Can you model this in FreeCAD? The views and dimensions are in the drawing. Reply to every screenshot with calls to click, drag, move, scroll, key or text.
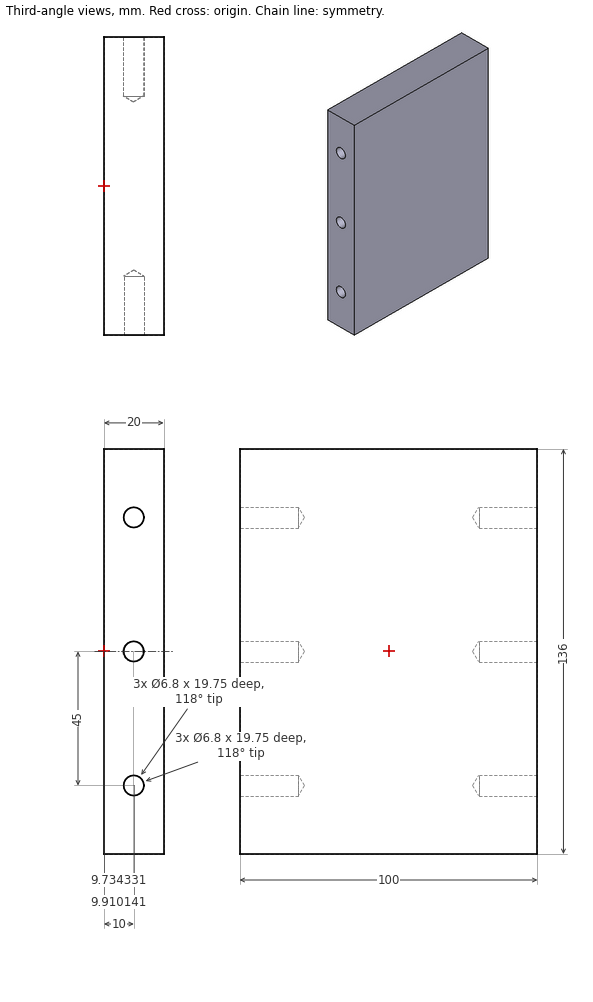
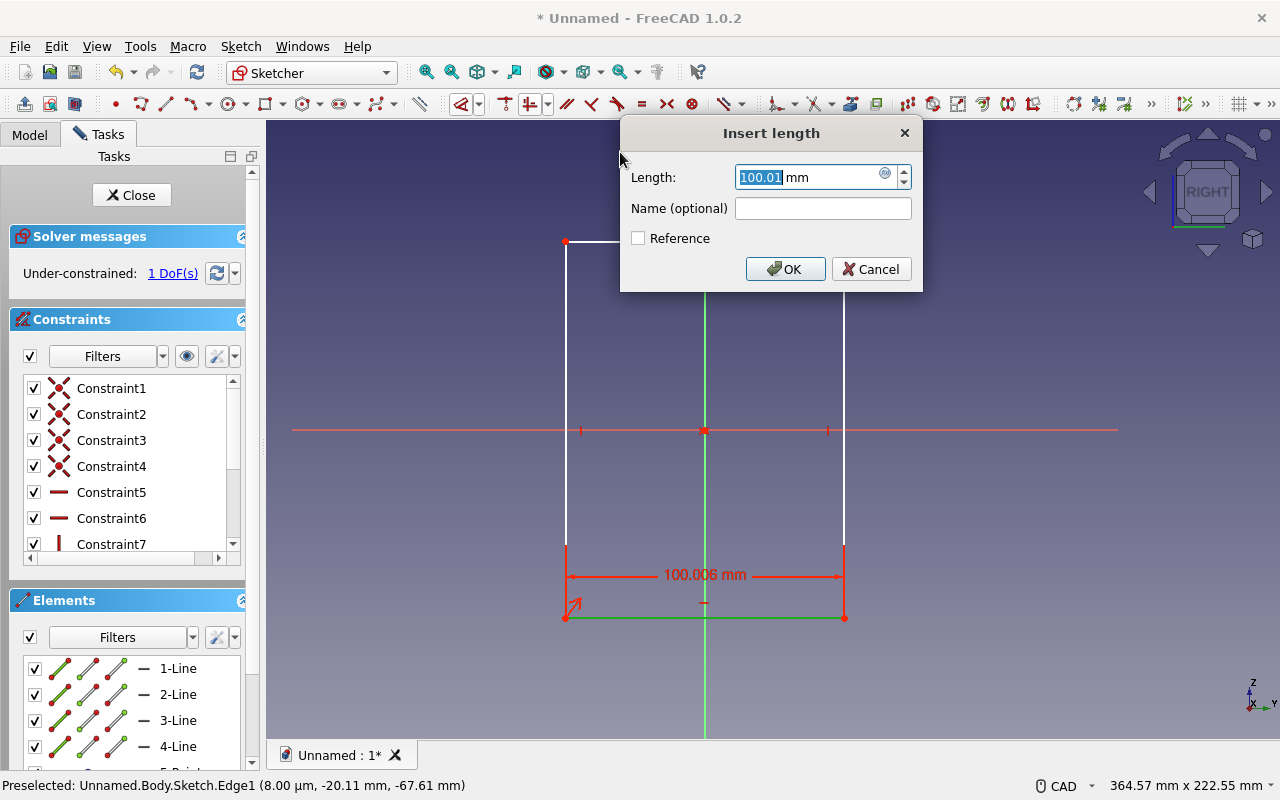
text(100)
key(Return)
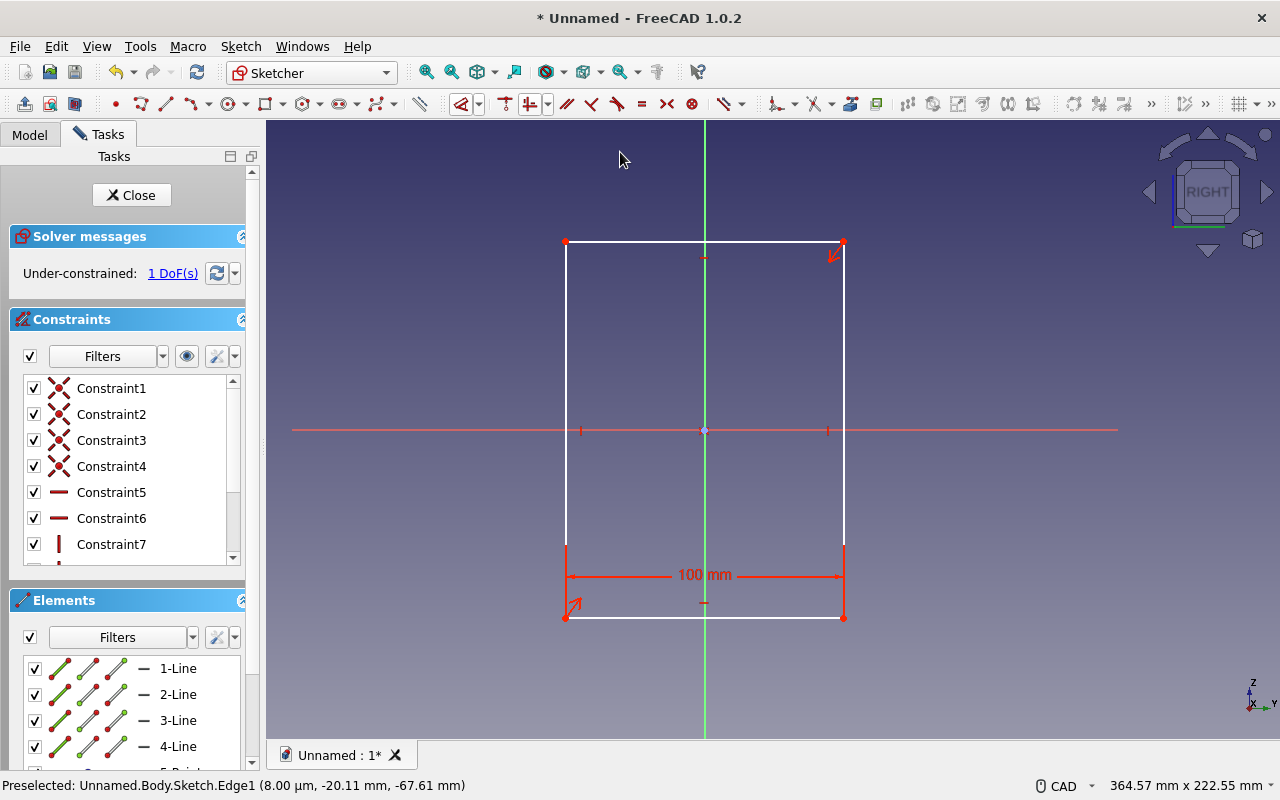
click(844, 505)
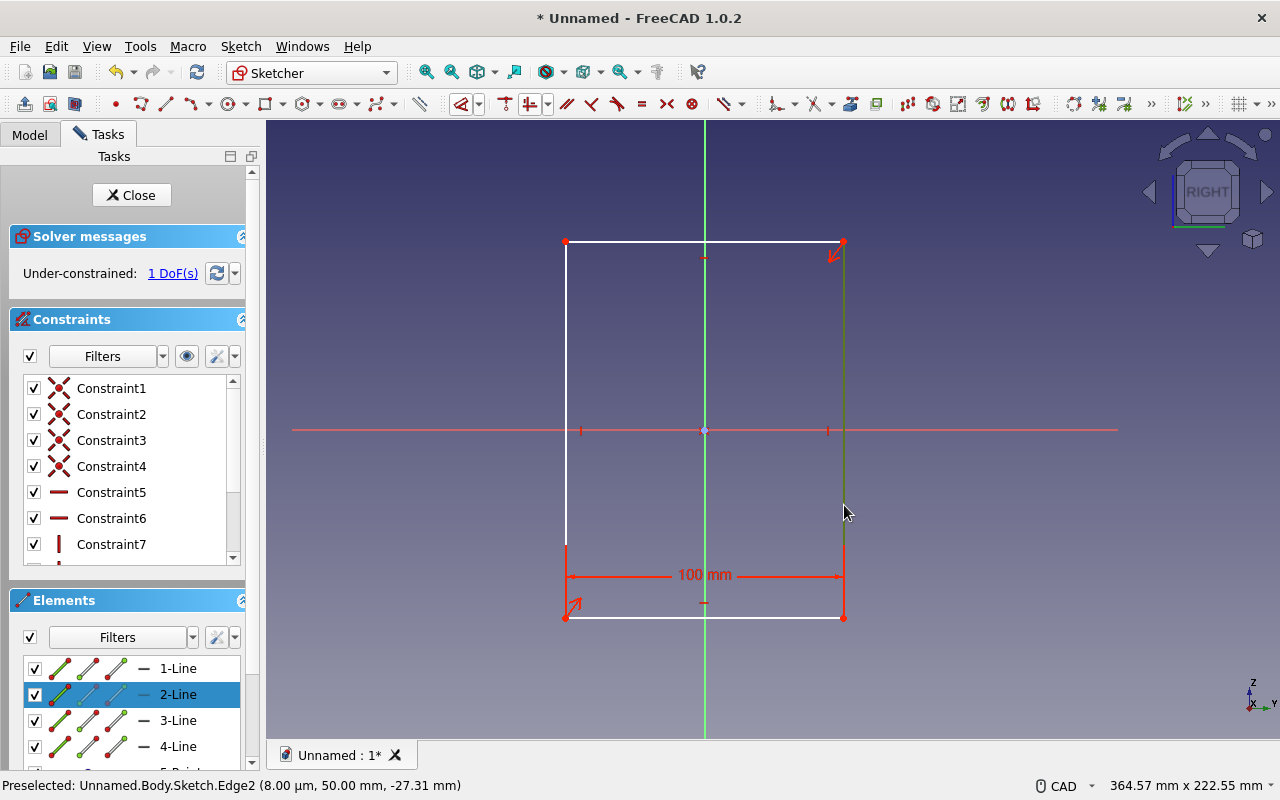
key(i)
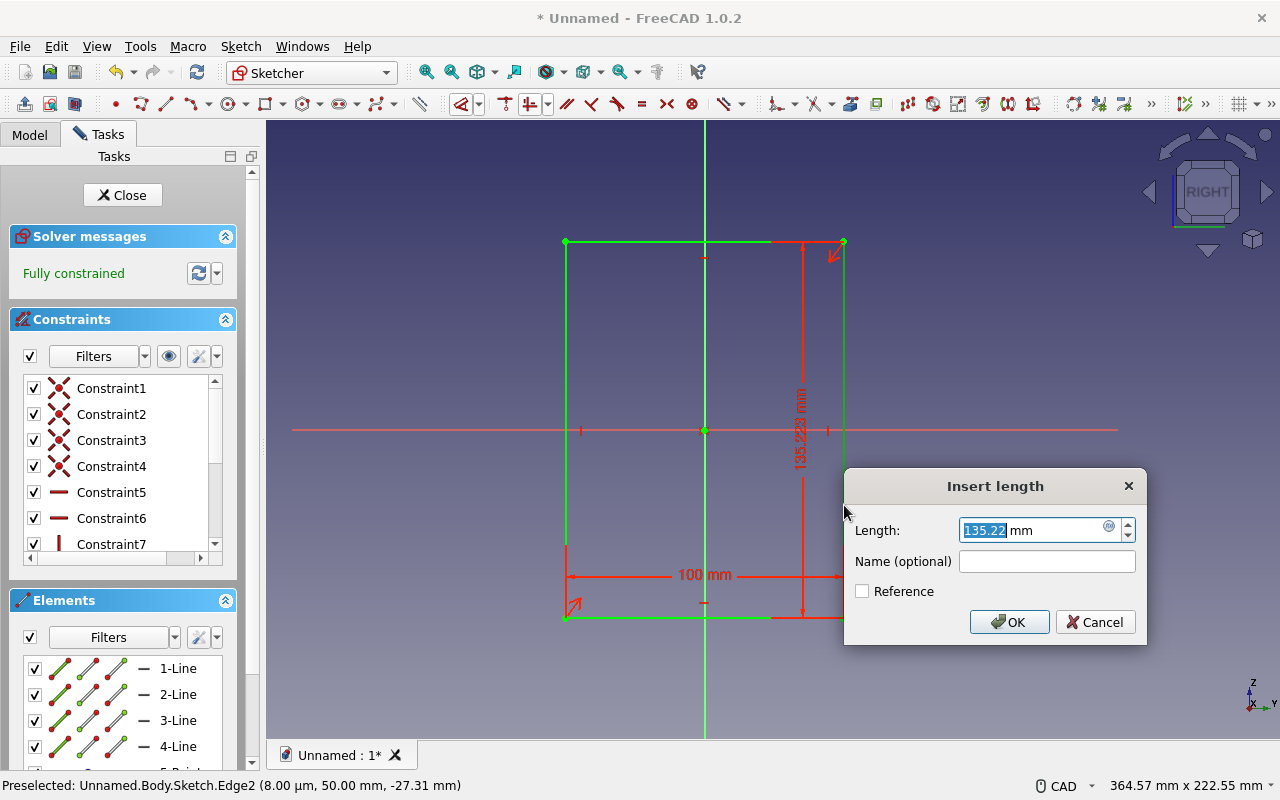
text(136)
key(Return)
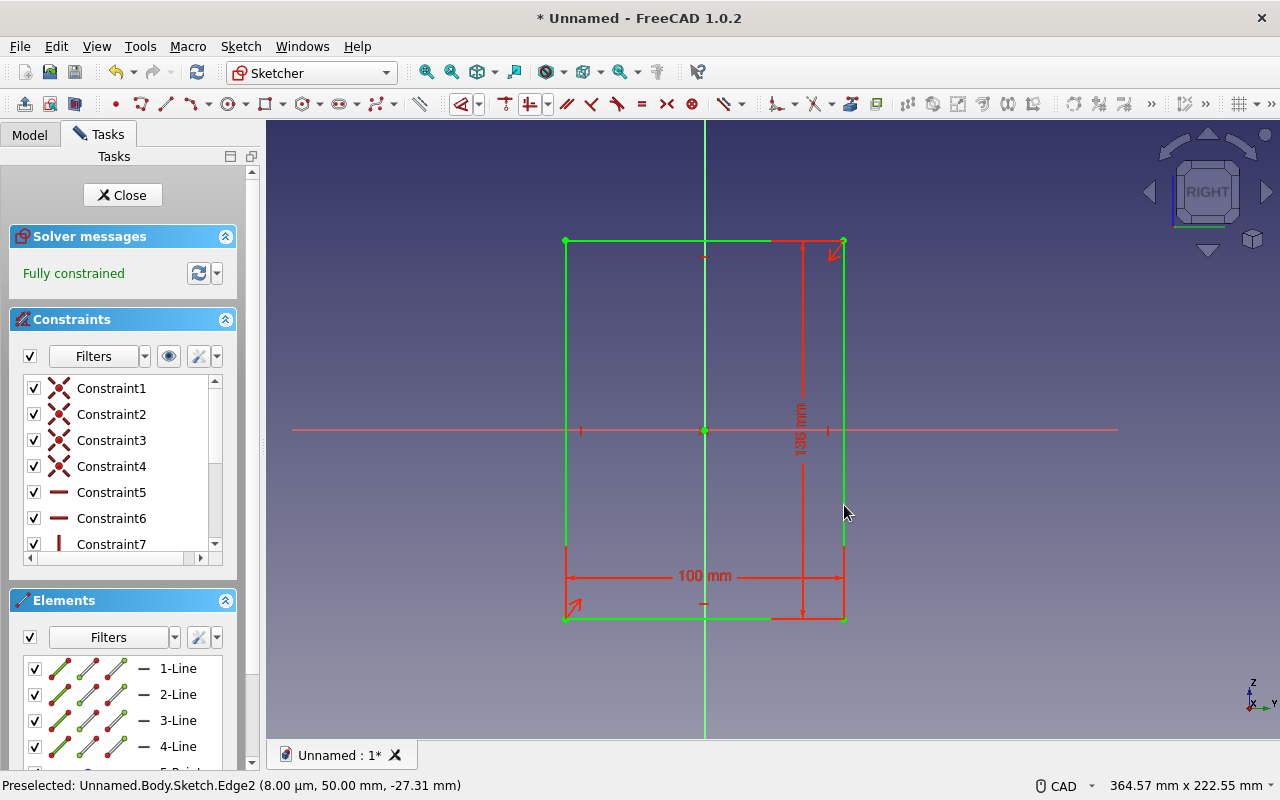
click(123, 195)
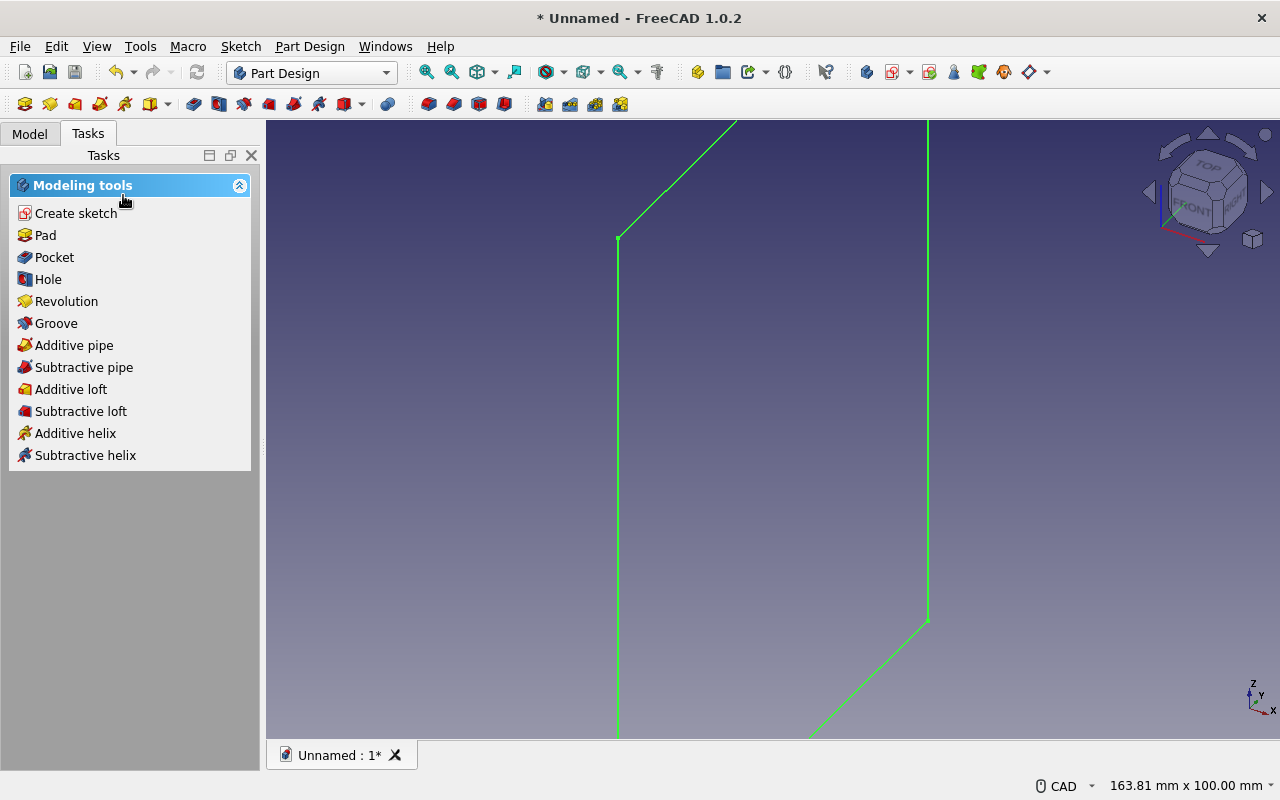
click(25, 104)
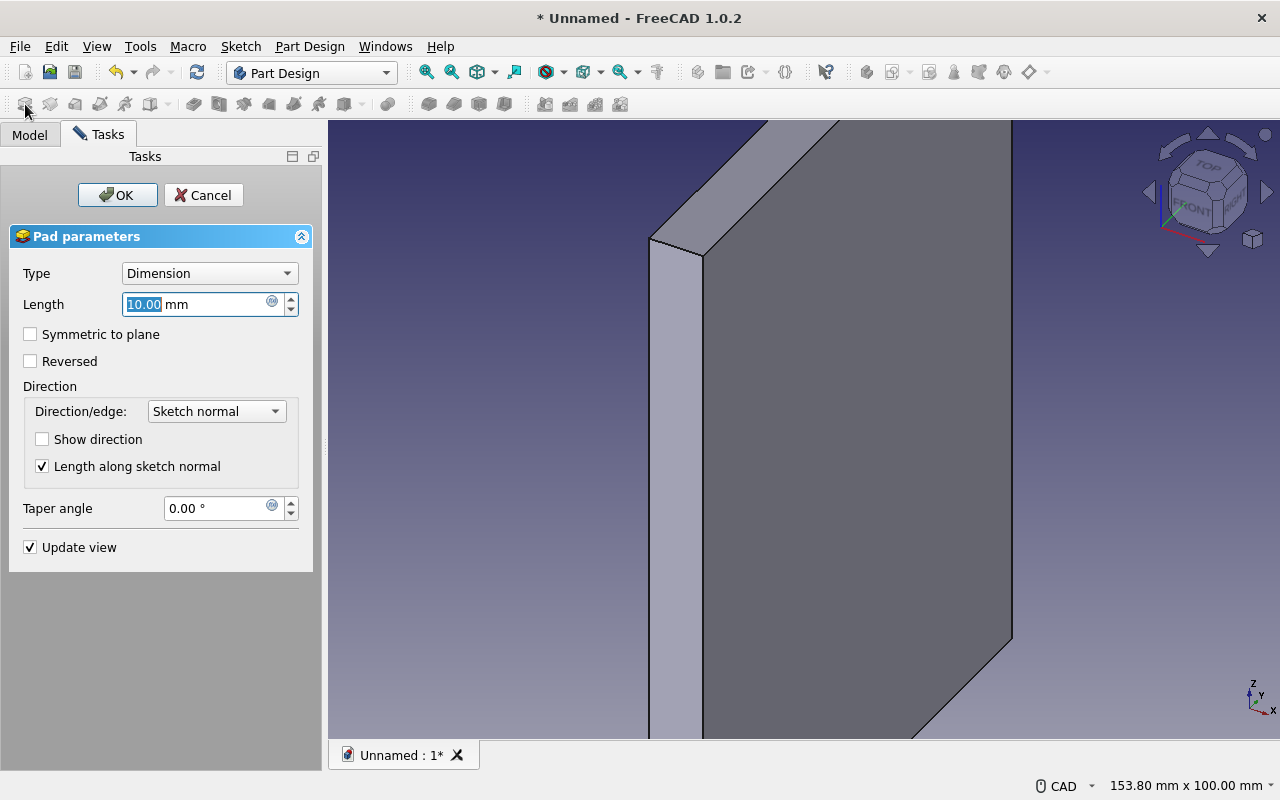
text(20)
key(Tab)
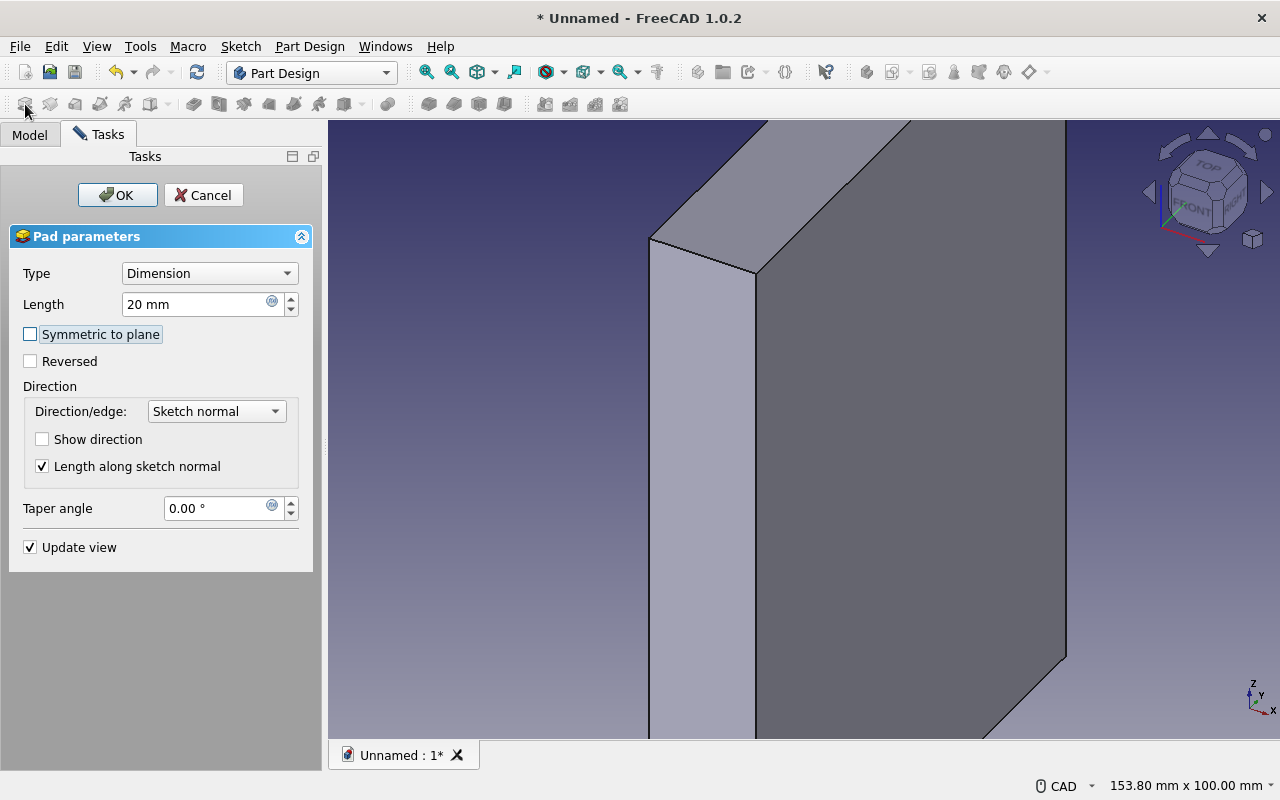
click(118, 195)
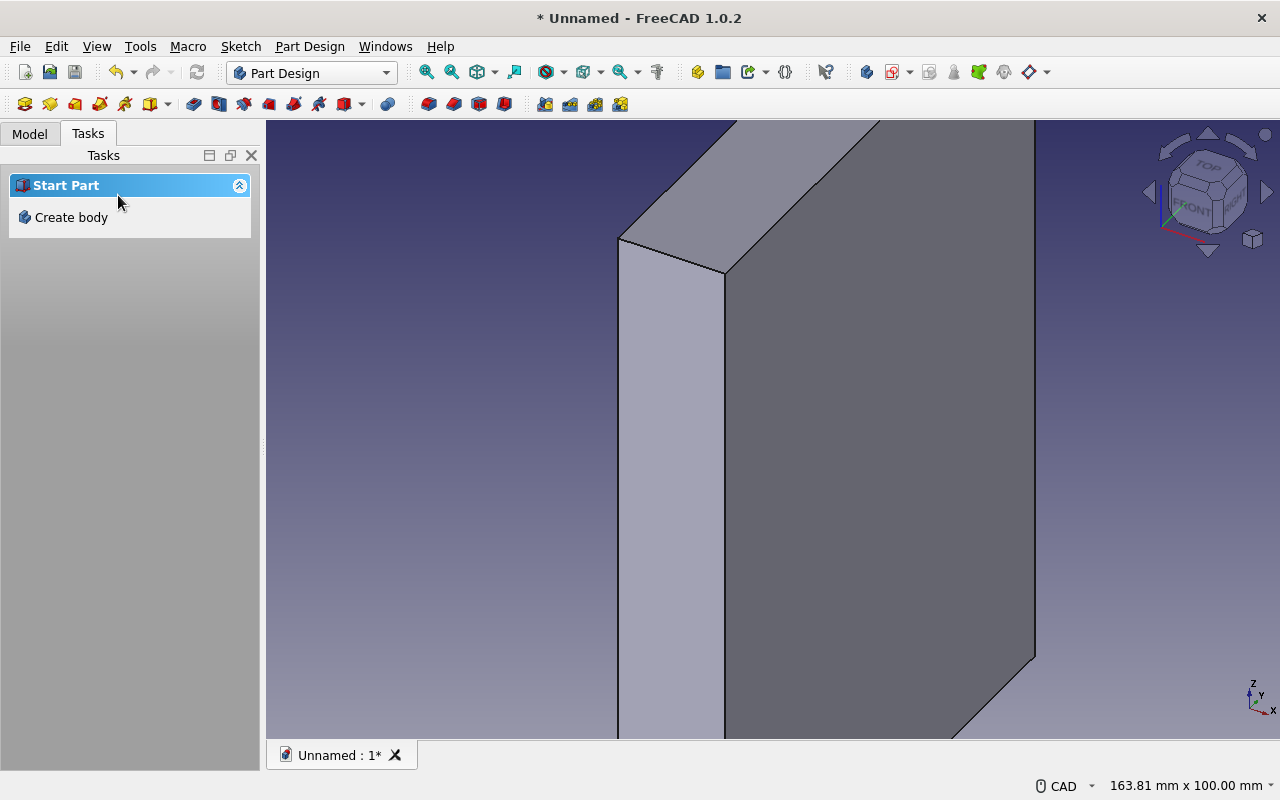
click(427, 72)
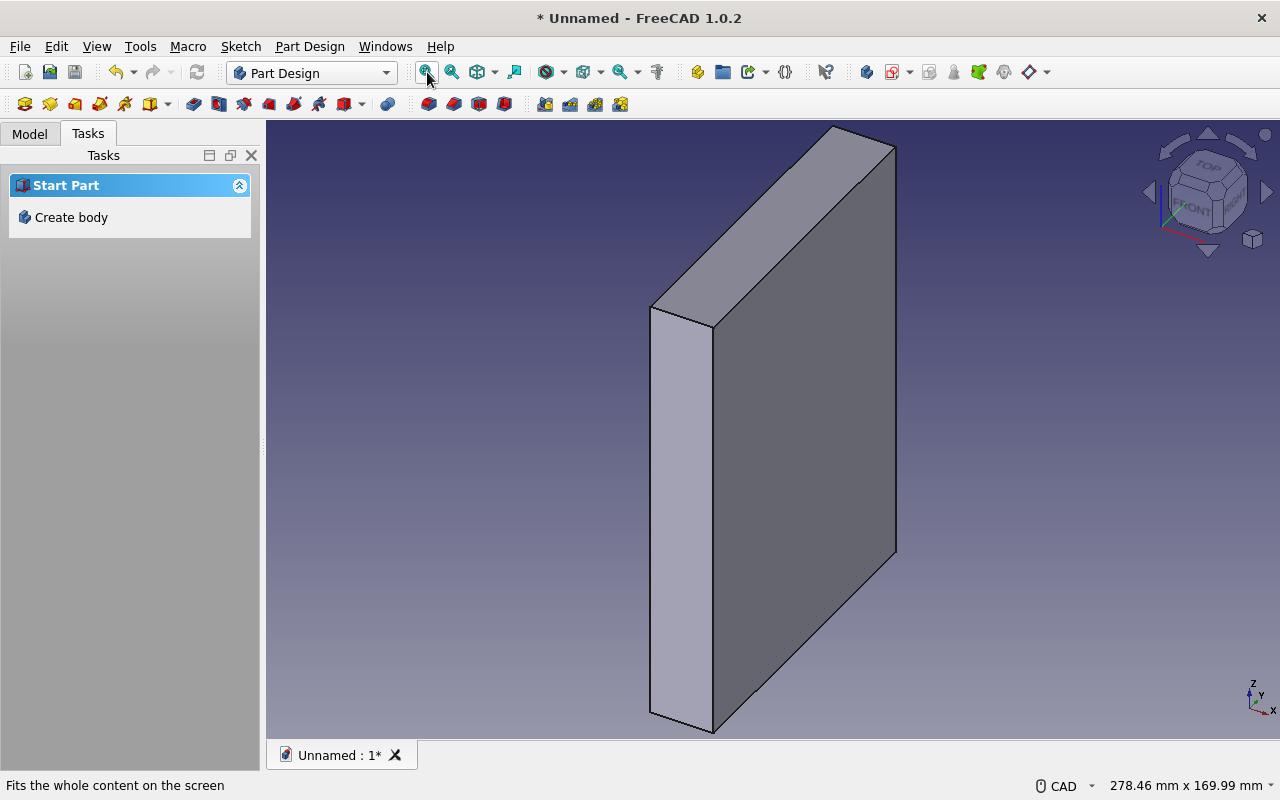
key(4)